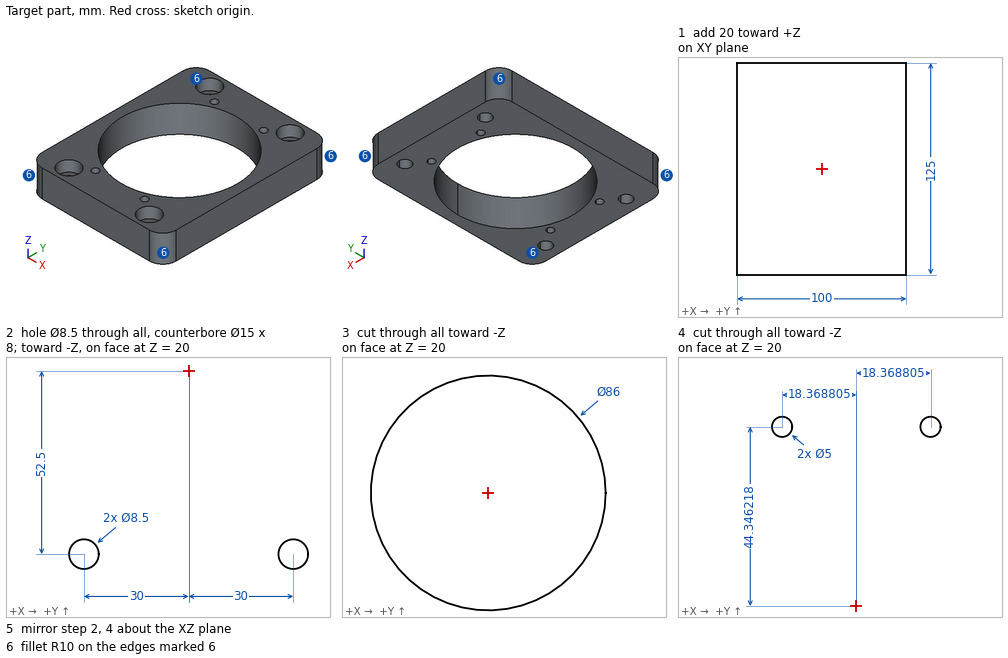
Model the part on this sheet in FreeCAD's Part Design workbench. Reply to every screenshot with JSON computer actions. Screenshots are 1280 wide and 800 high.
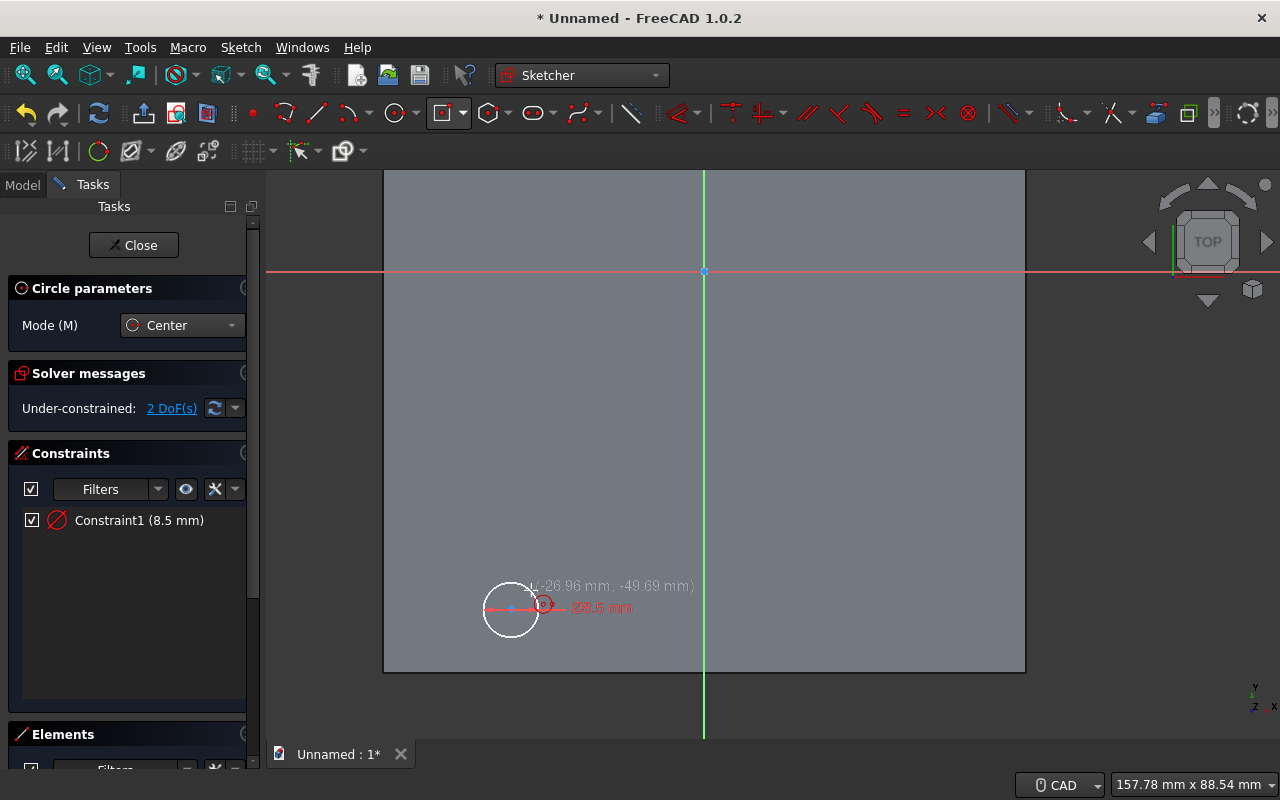
{"action": "left_click", "coordinate": [897, 609]}
{"action": "mouse_move", "coordinate": [916, 590]}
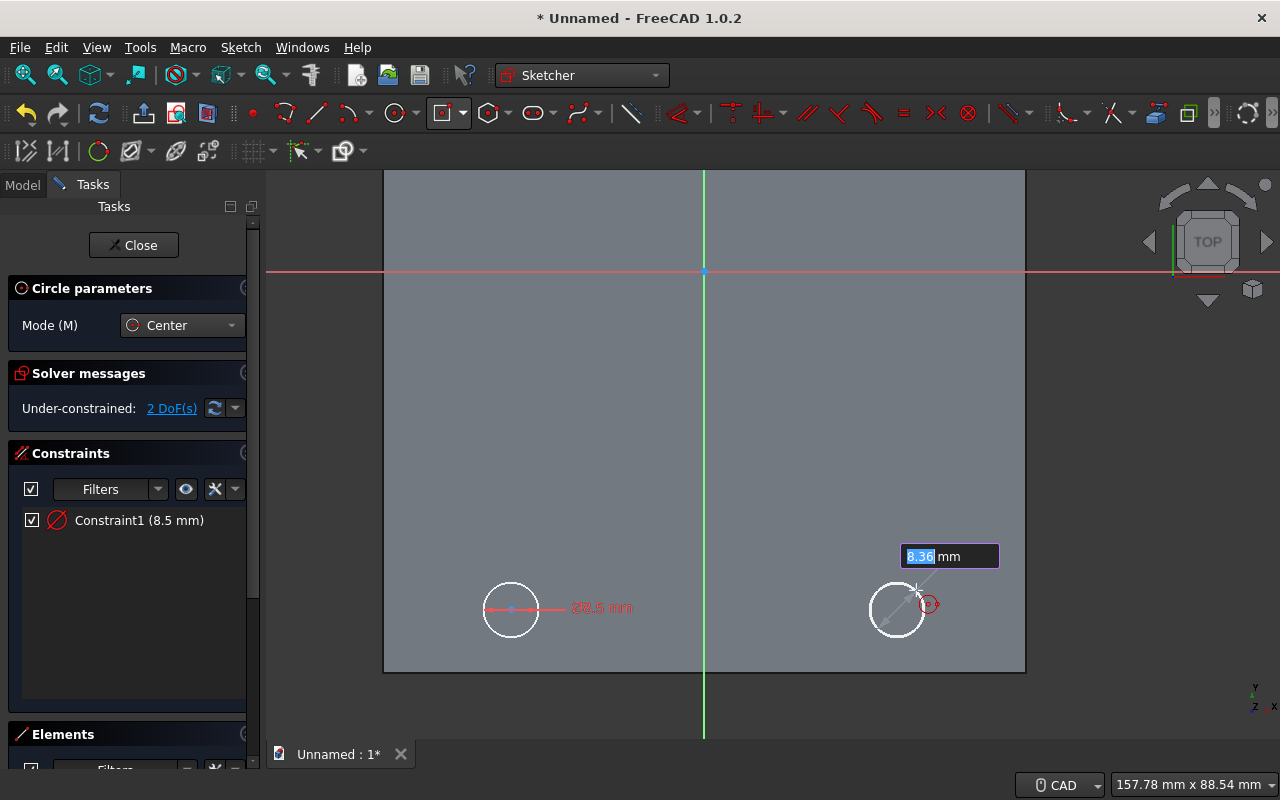
{"action": "type", "text": "8.5"}
{"action": "key", "text": "Return"}
{"action": "key", "text": "Escape"}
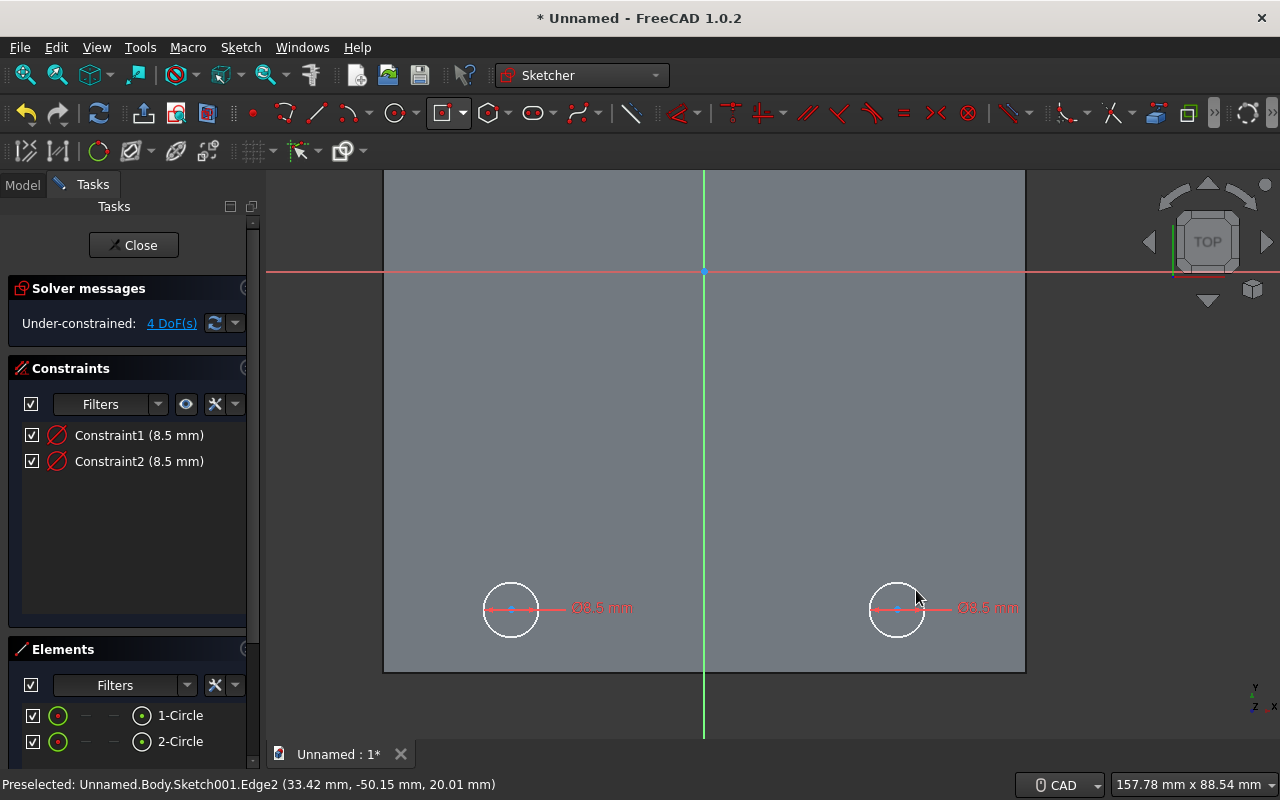
{"action": "left_click", "coordinate": [511, 610]}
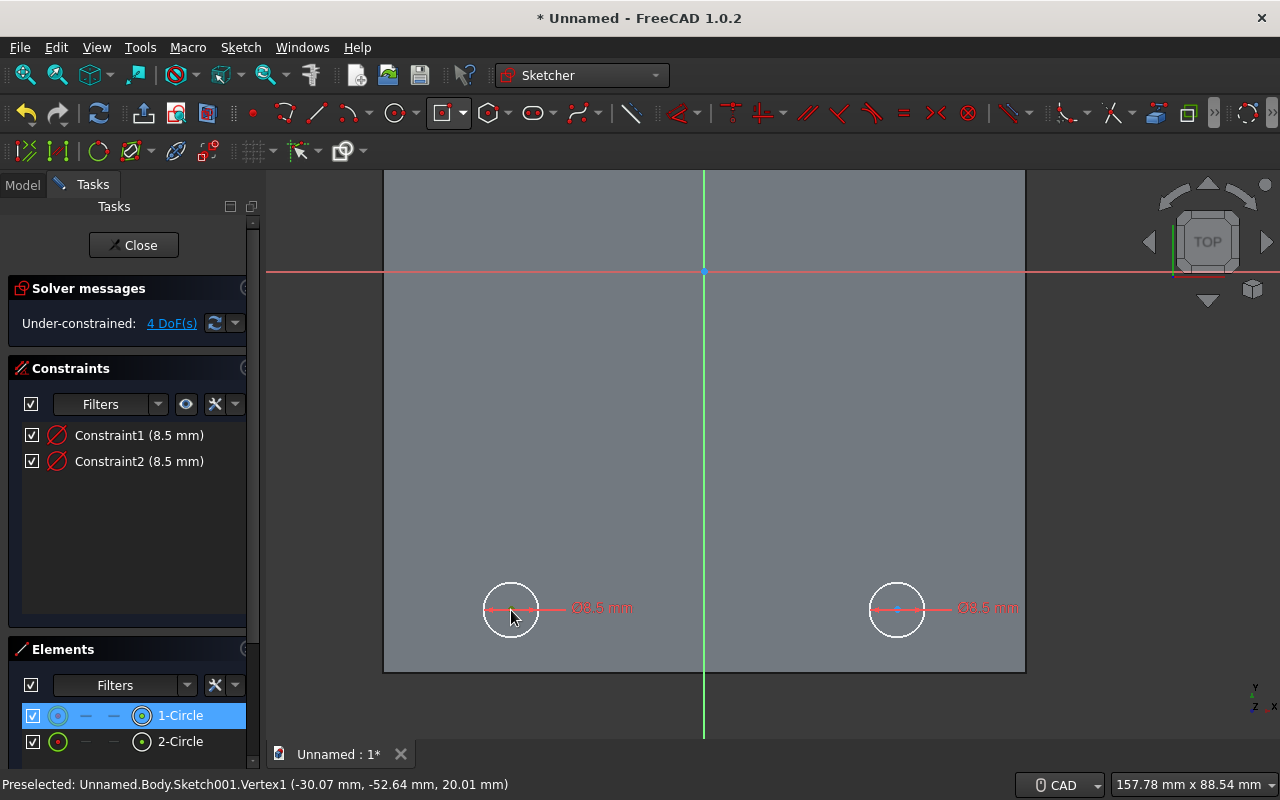
{"action": "left_click", "coordinate": [897, 610]}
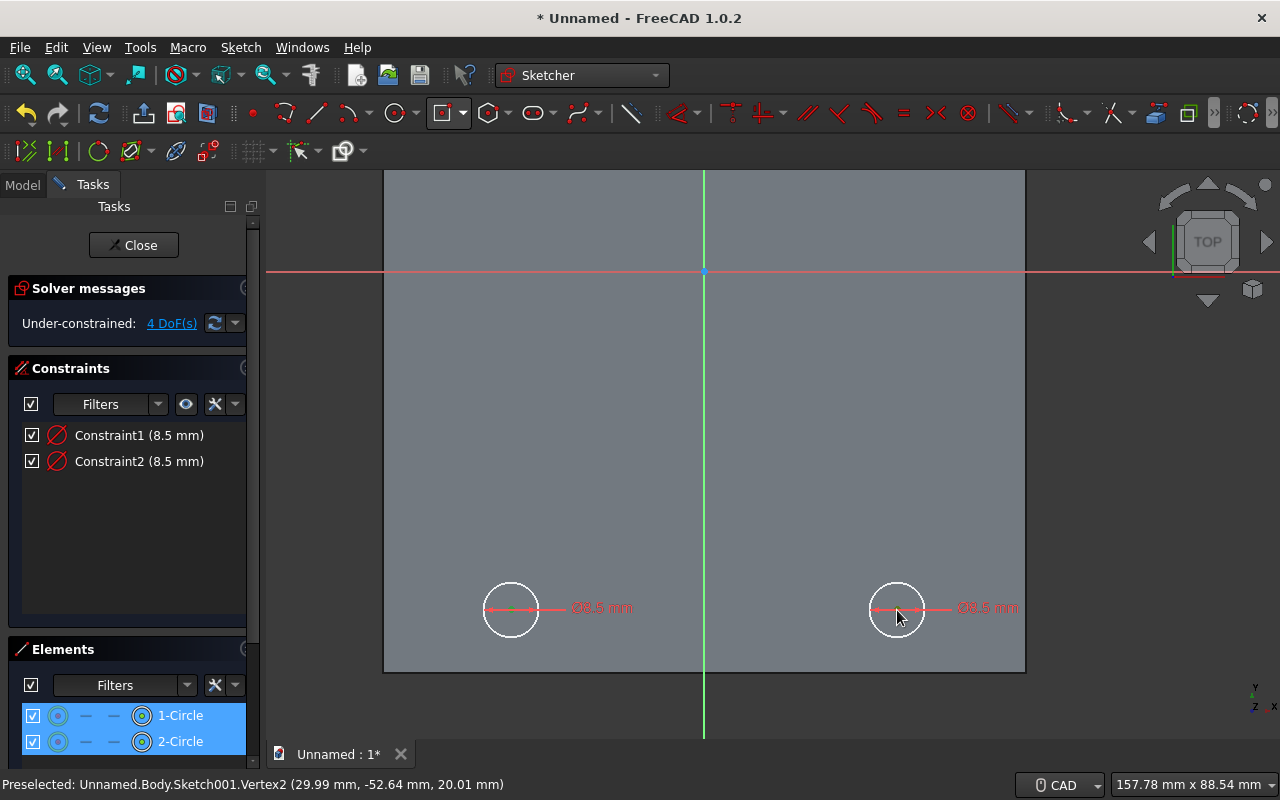
{"action": "left_click", "coordinate": [786, 114]}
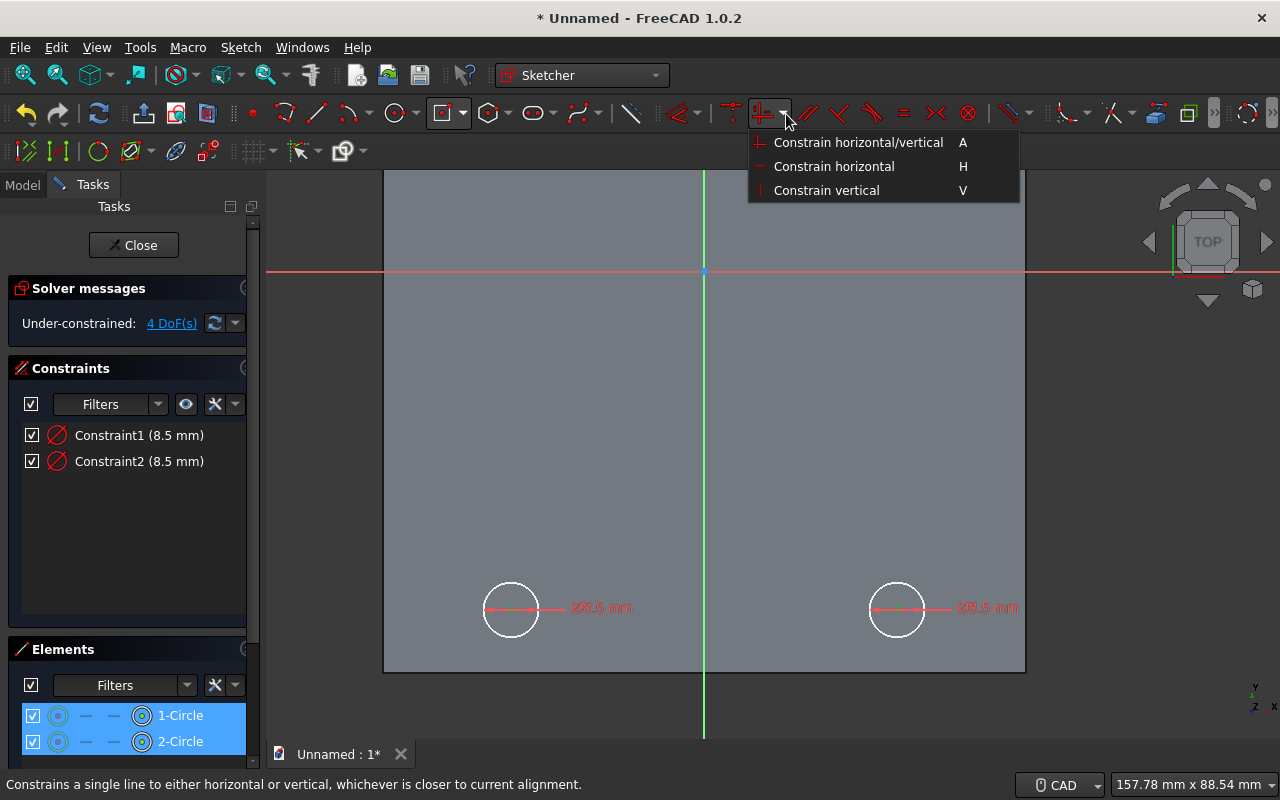
{"action": "left_click", "coordinate": [884, 166]}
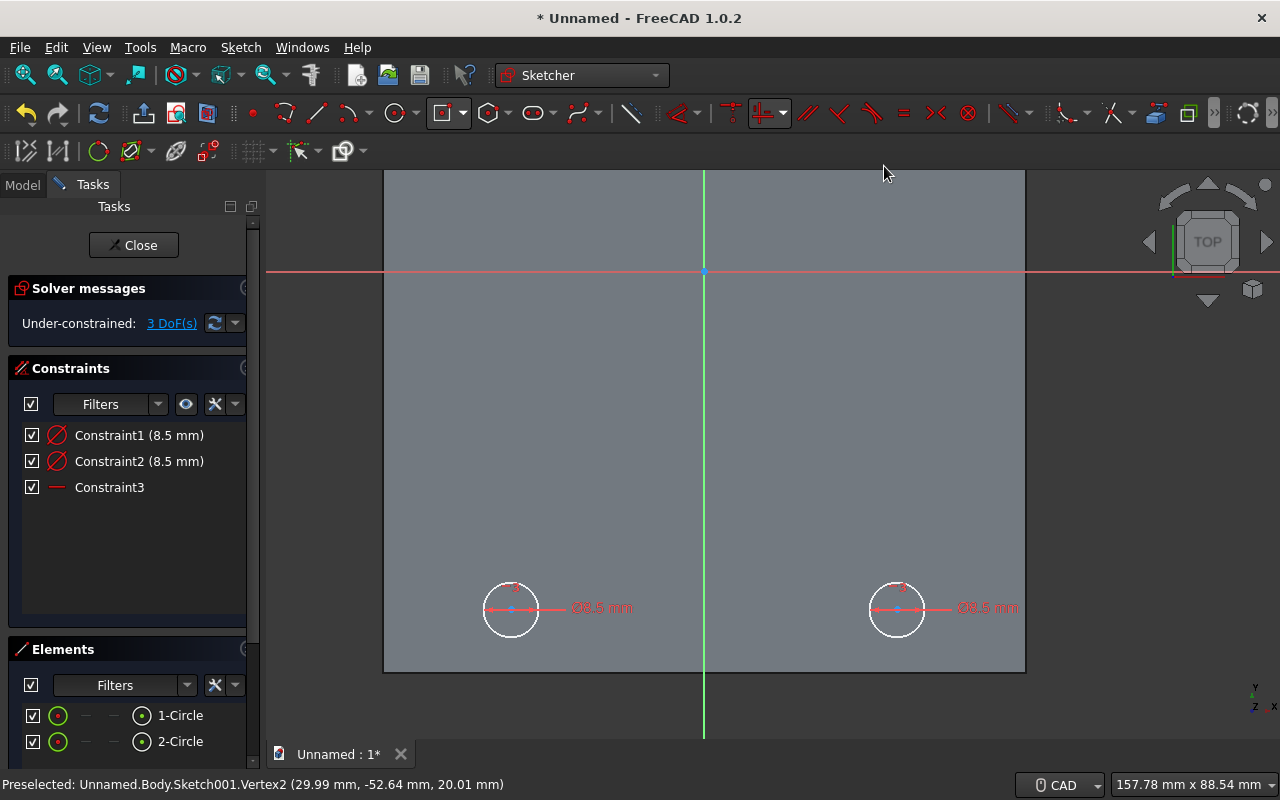
{"action": "left_click", "coordinate": [678, 114]}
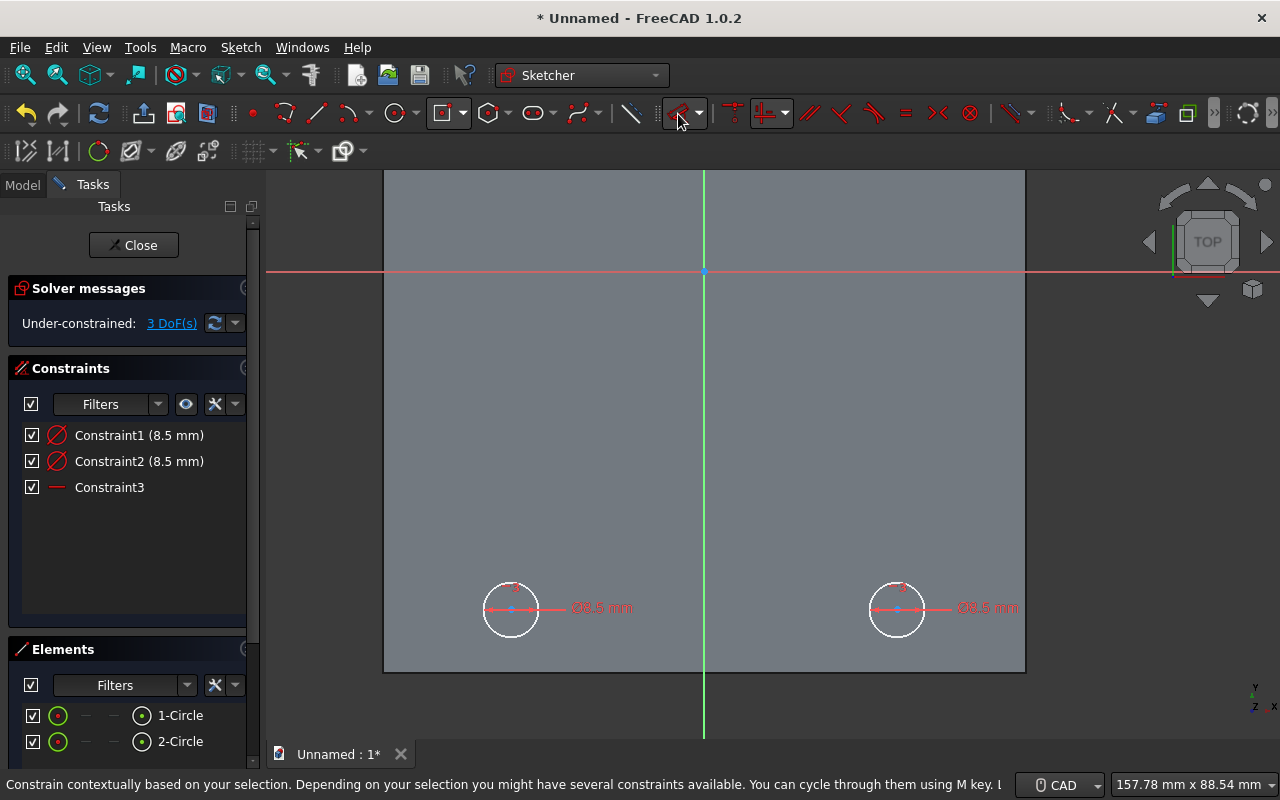
{"action": "left_click", "coordinate": [511, 610]}
{"action": "left_click", "coordinate": [608, 238]}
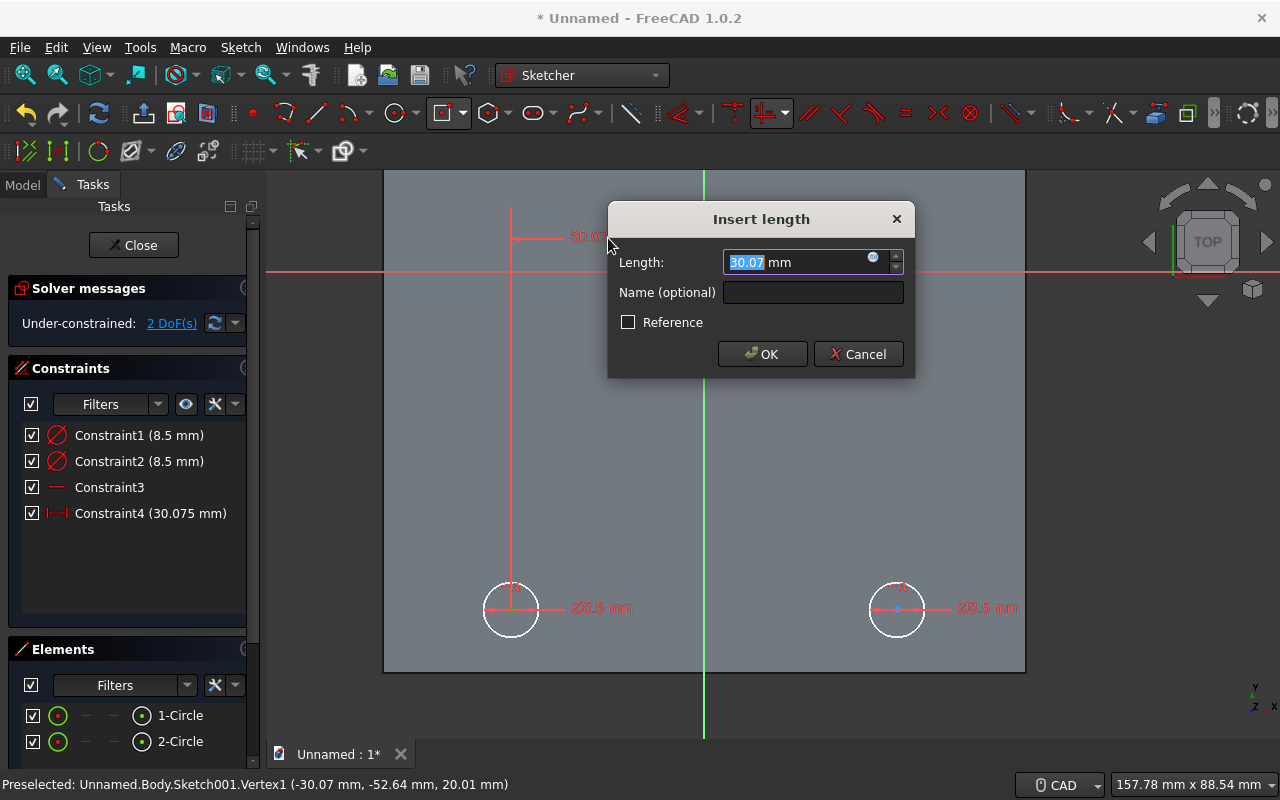
{"action": "type", "text": "30"}
{"action": "key", "text": "Return"}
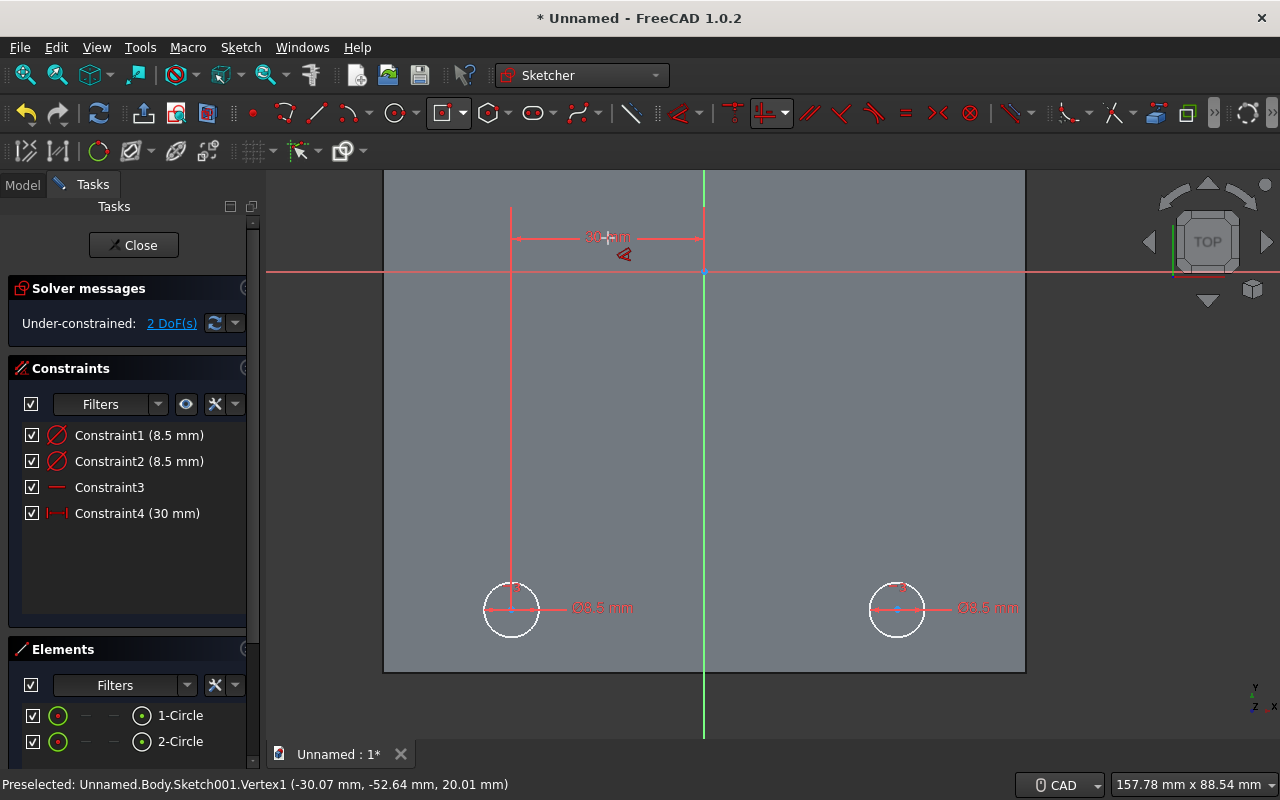
{"action": "left_click", "coordinate": [897, 610]}
{"action": "left_click", "coordinate": [801, 238]}